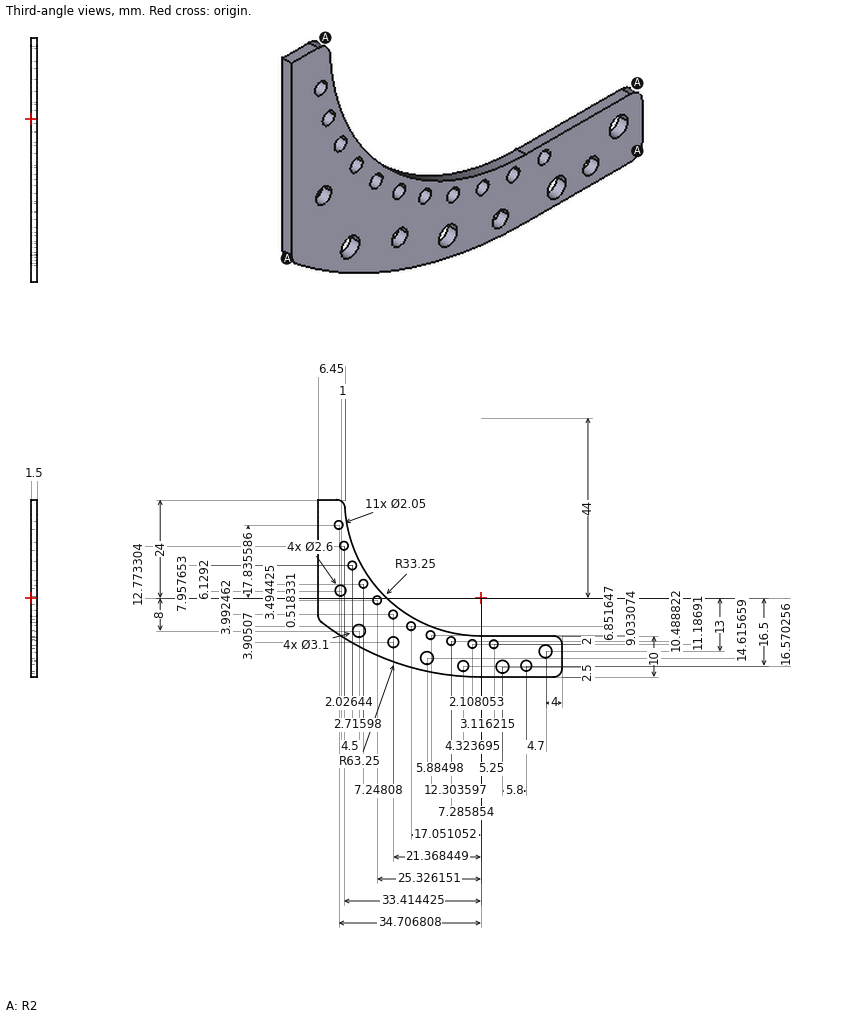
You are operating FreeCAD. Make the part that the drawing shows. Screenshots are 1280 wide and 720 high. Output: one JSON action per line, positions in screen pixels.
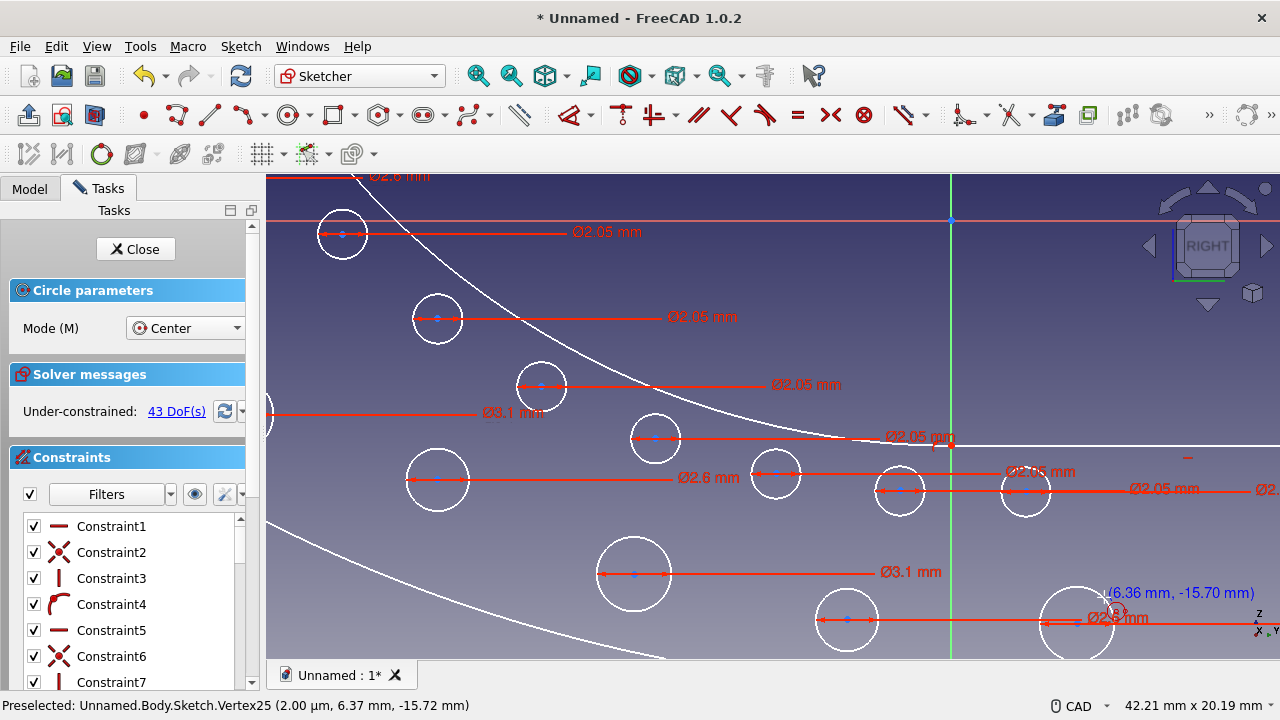
{"action": "scroll", "coordinate": [701, 525], "scroll_direction": "down", "scroll_amount": 6}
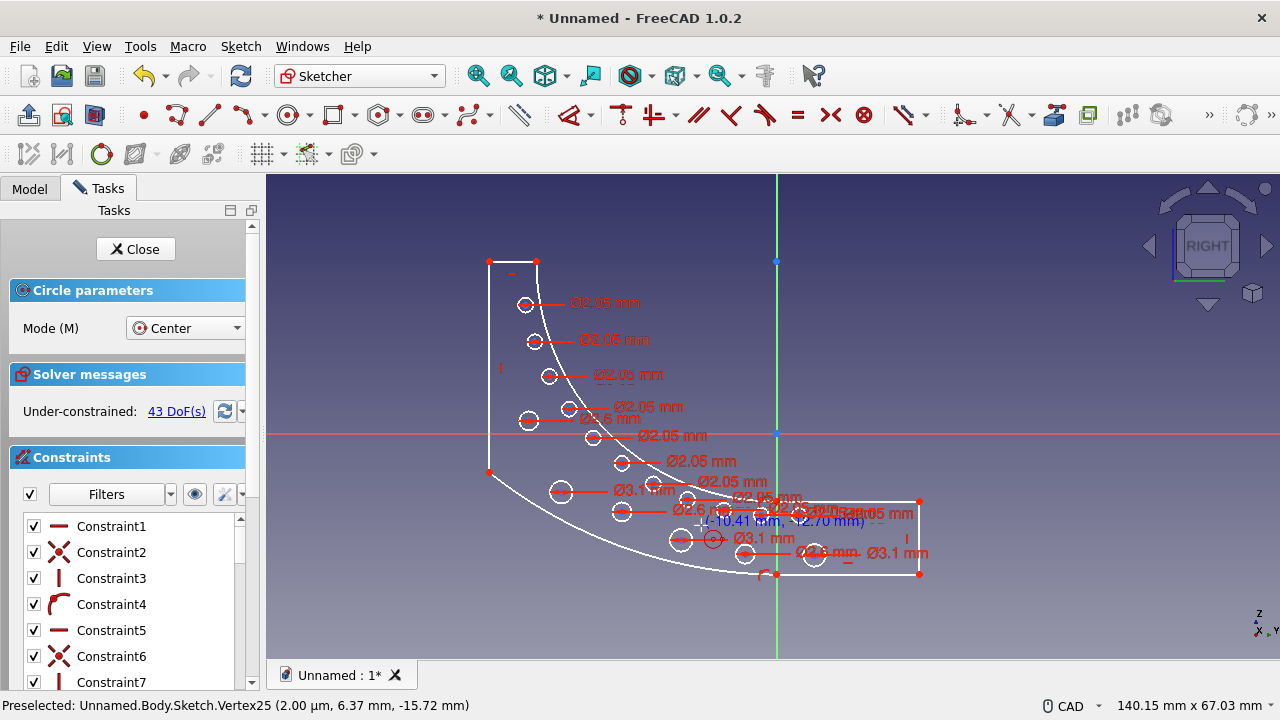
{"action": "scroll", "coordinate": [891, 528], "scroll_direction": "up", "scroll_amount": 4}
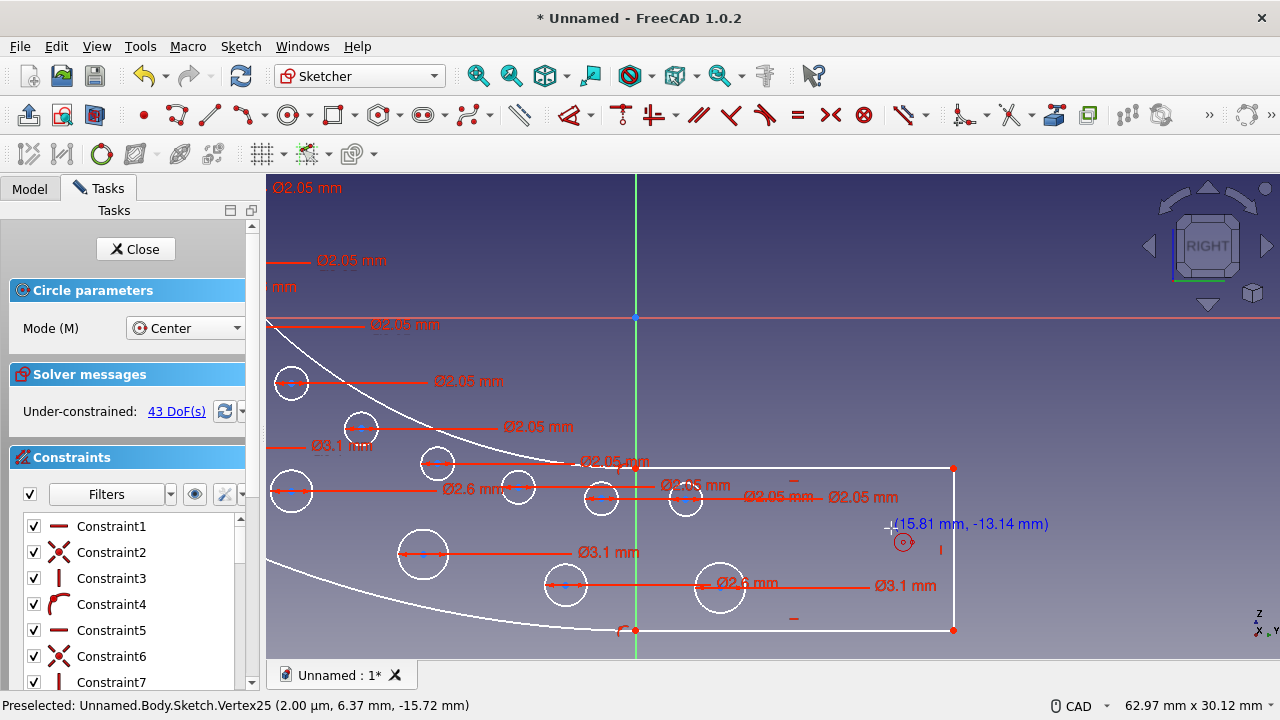
{"action": "left_click", "coordinate": [889, 527]}
{"action": "mouse_move", "coordinate": [907, 509]}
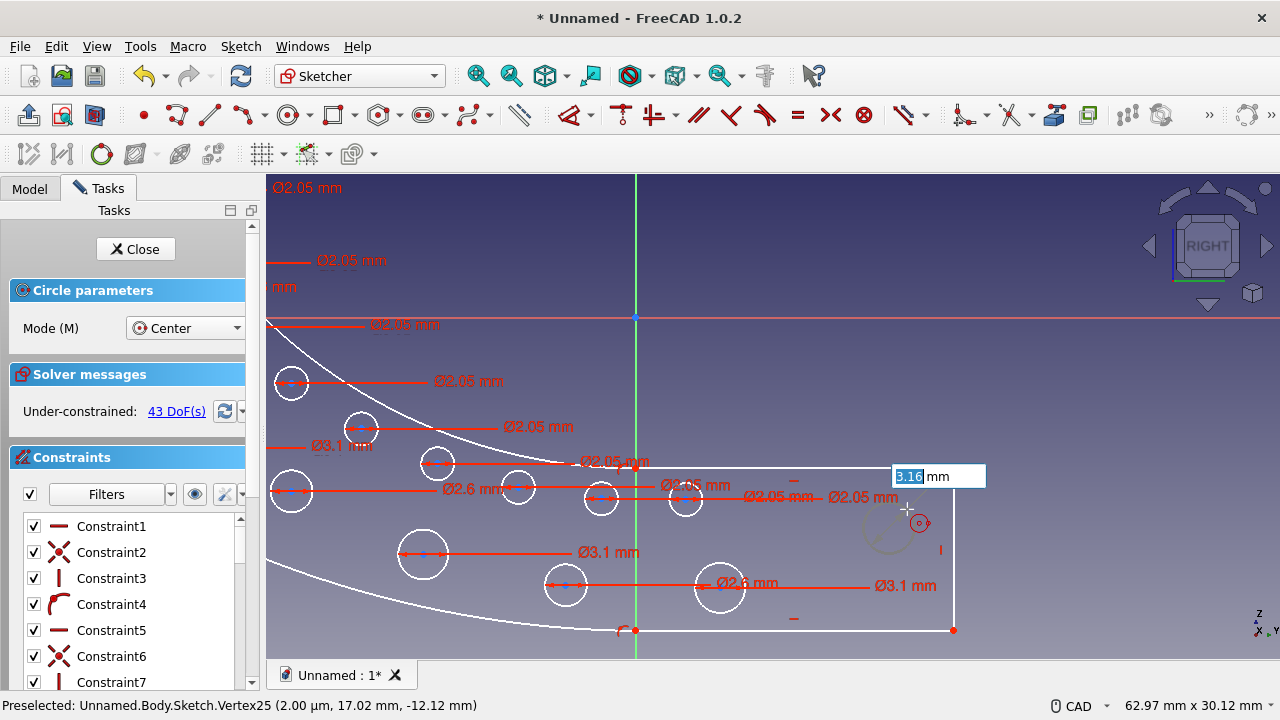
{"action": "type", "text": "3.1"}
{"action": "key", "text": "Return"}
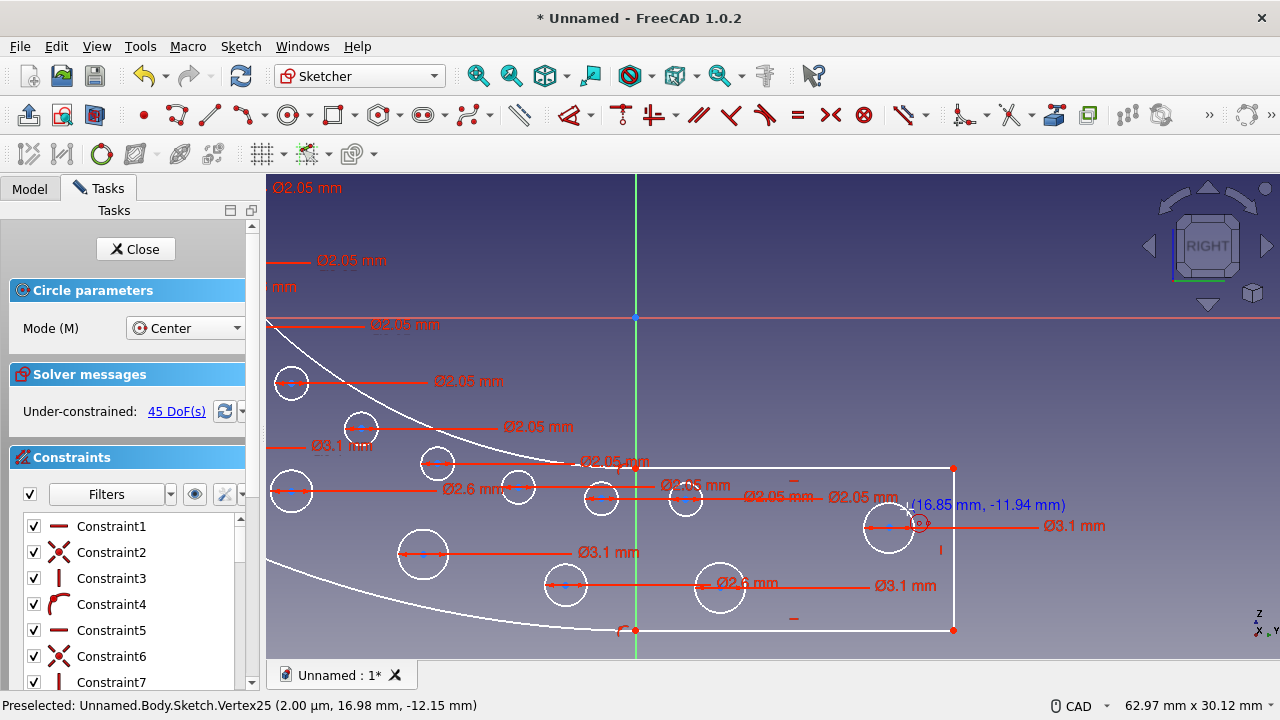
{"action": "left_click", "coordinate": [814, 583]}
{"action": "mouse_move", "coordinate": [828, 569]}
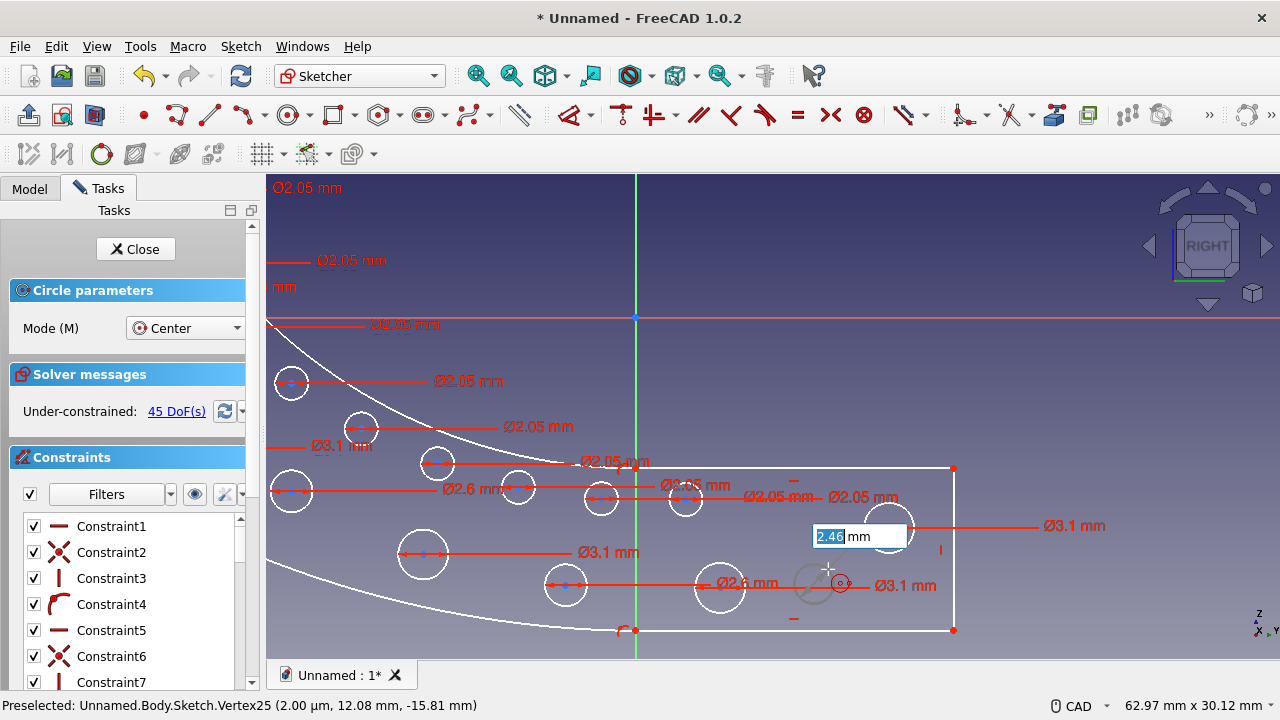
{"action": "type", "text": "2.6"}
{"action": "key", "text": "Return"}
{"action": "key", "text": "Escape"}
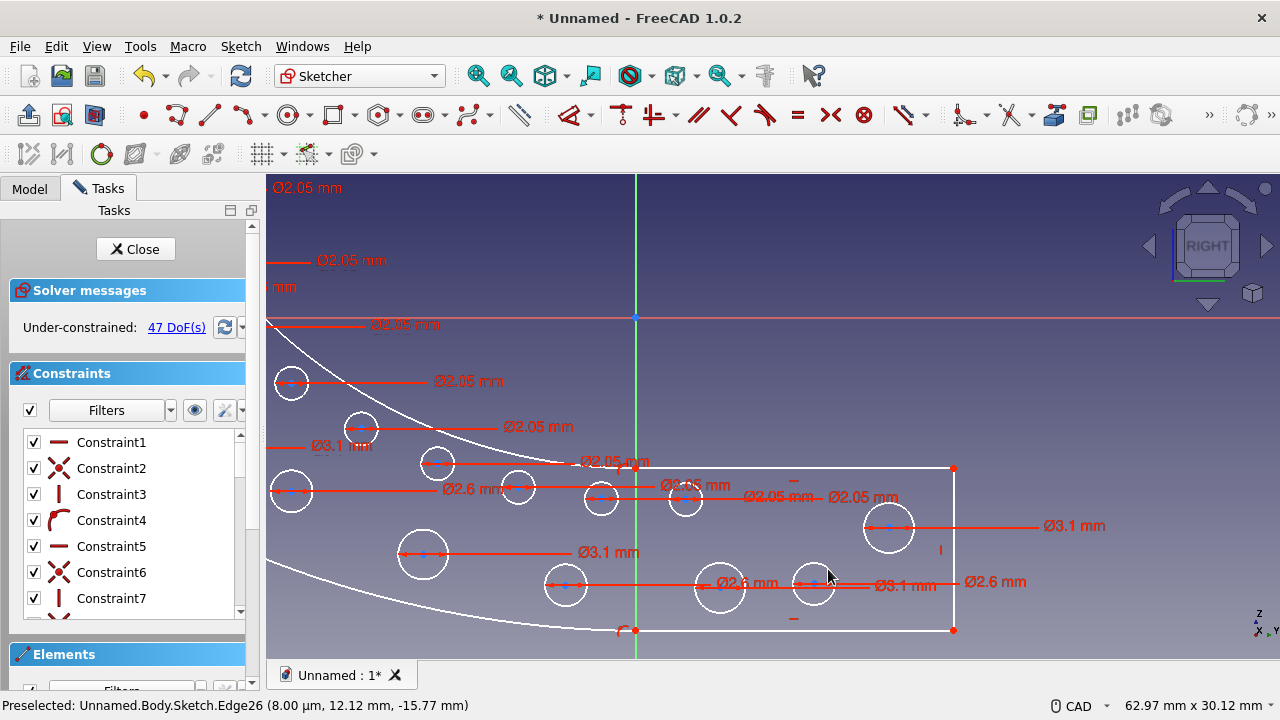
{"action": "scroll", "coordinate": [892, 528], "scroll_direction": "down", "scroll_amount": 4}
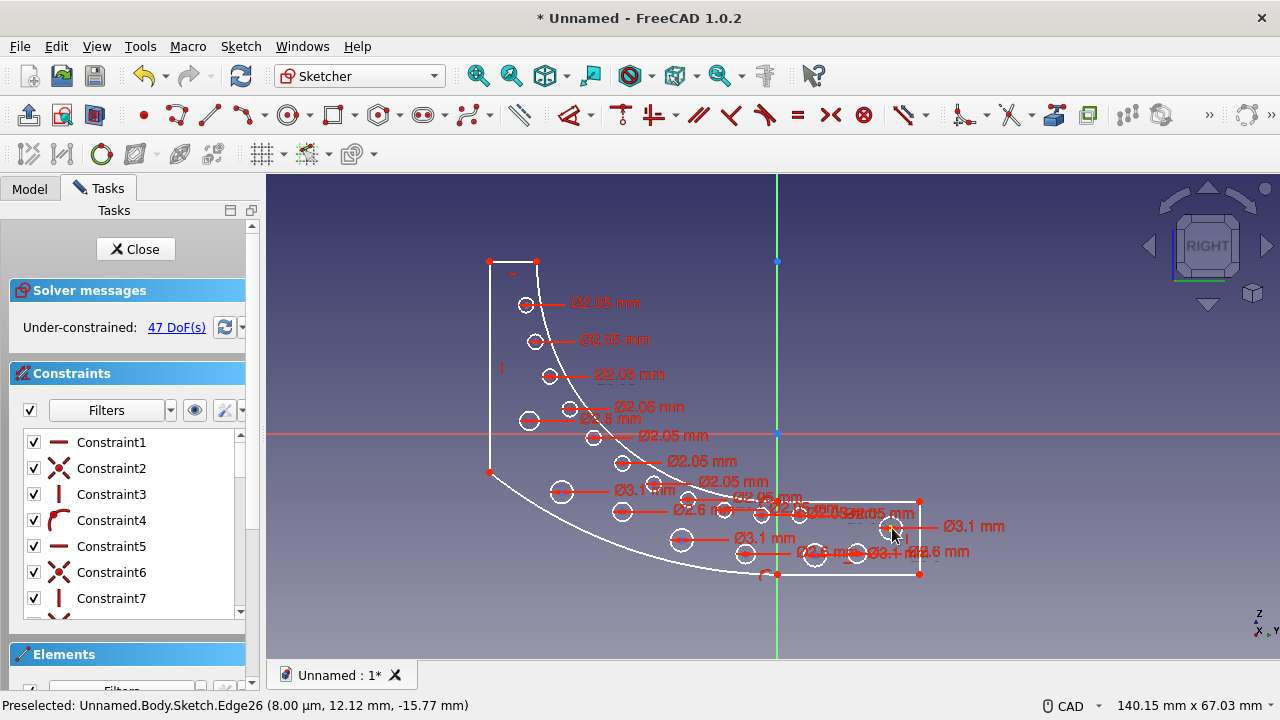
{"action": "scroll", "coordinate": [703, 572], "scroll_direction": "down", "scroll_amount": 2}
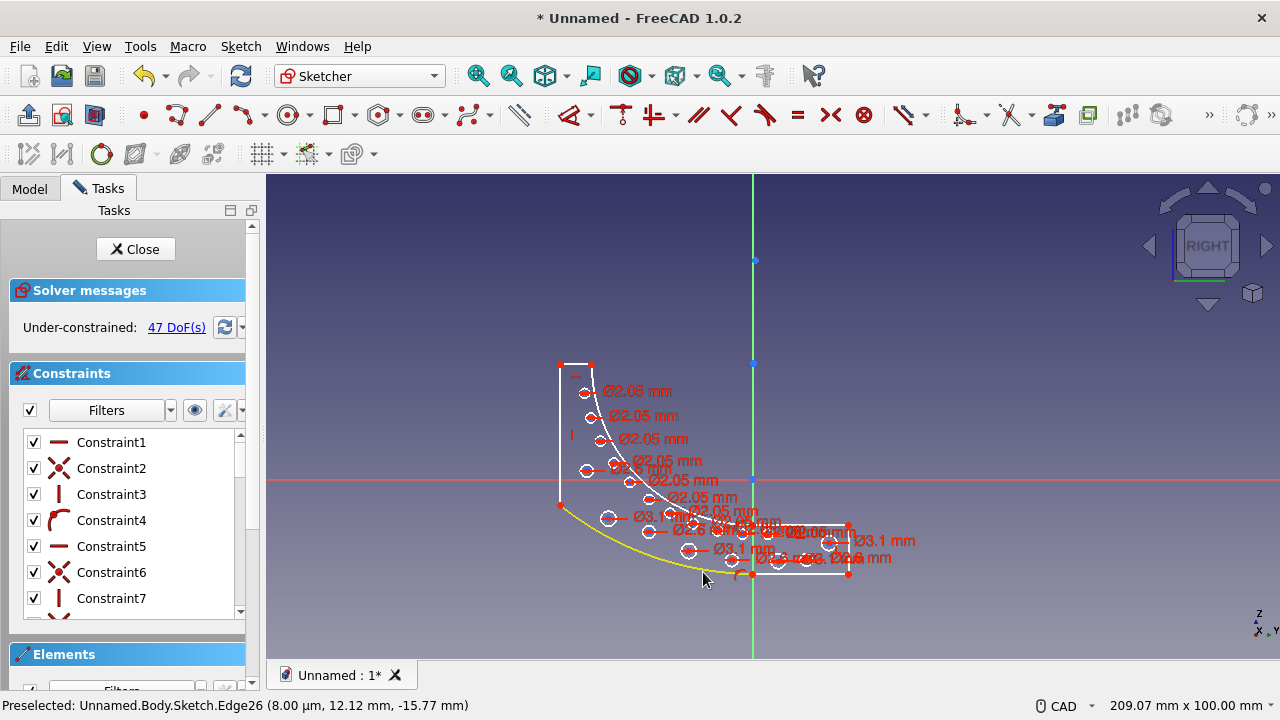
{"action": "left_click", "coordinate": [756, 260]}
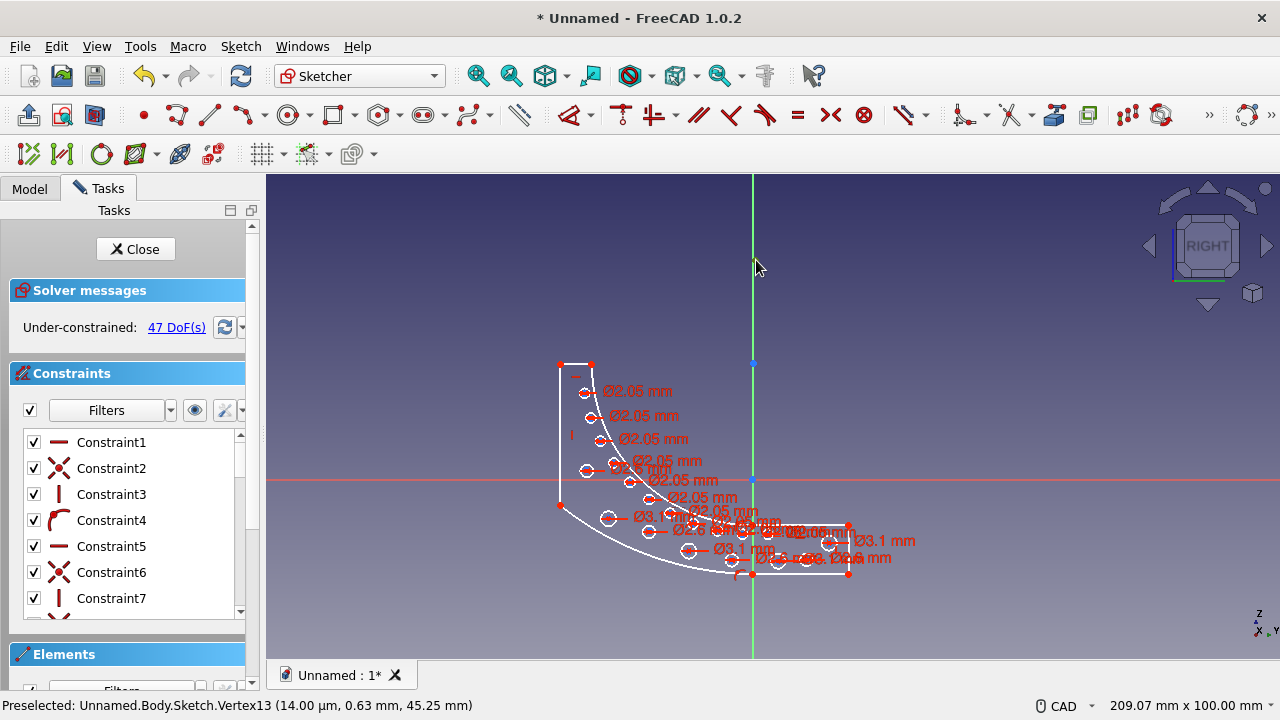
{"action": "left_click", "coordinate": [753, 447]}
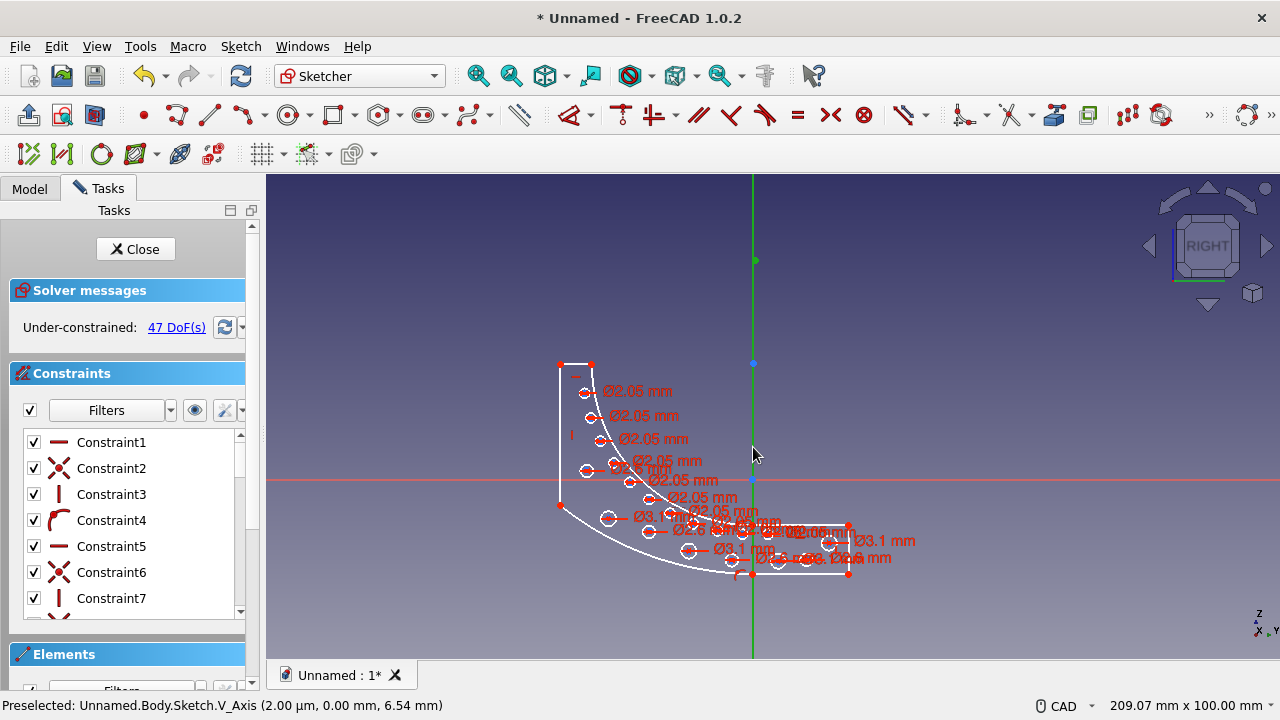
{"action": "left_click", "coordinate": [621, 116]}